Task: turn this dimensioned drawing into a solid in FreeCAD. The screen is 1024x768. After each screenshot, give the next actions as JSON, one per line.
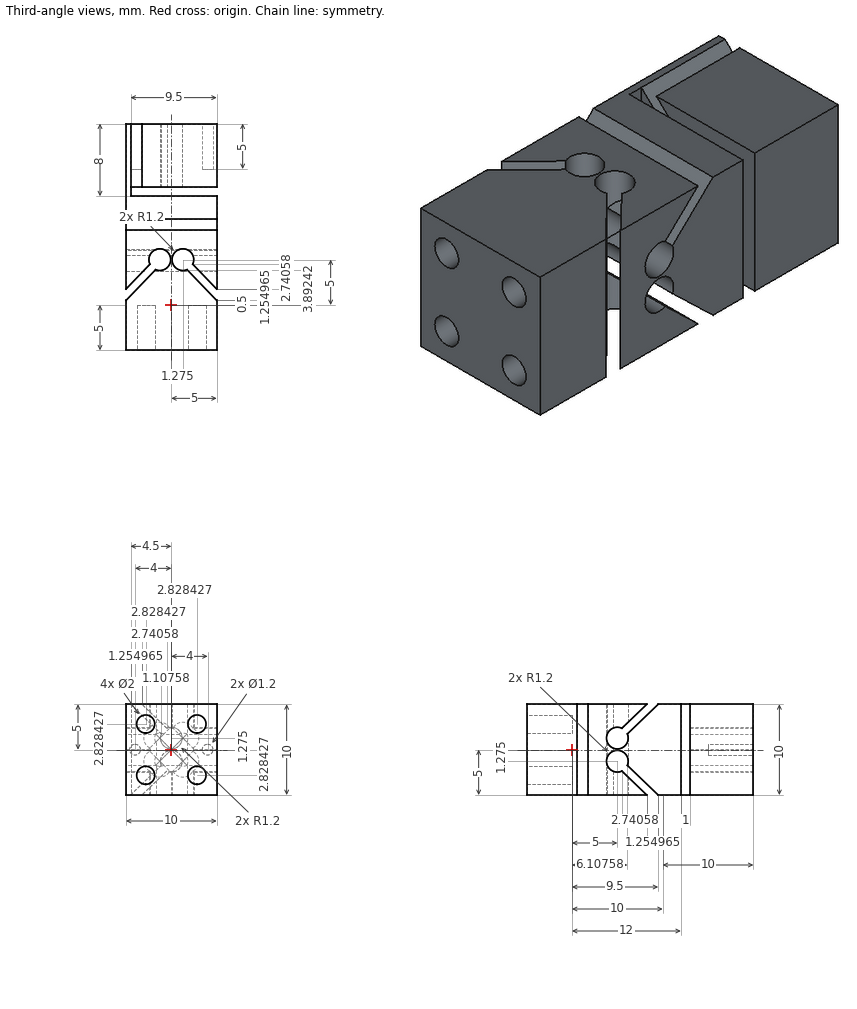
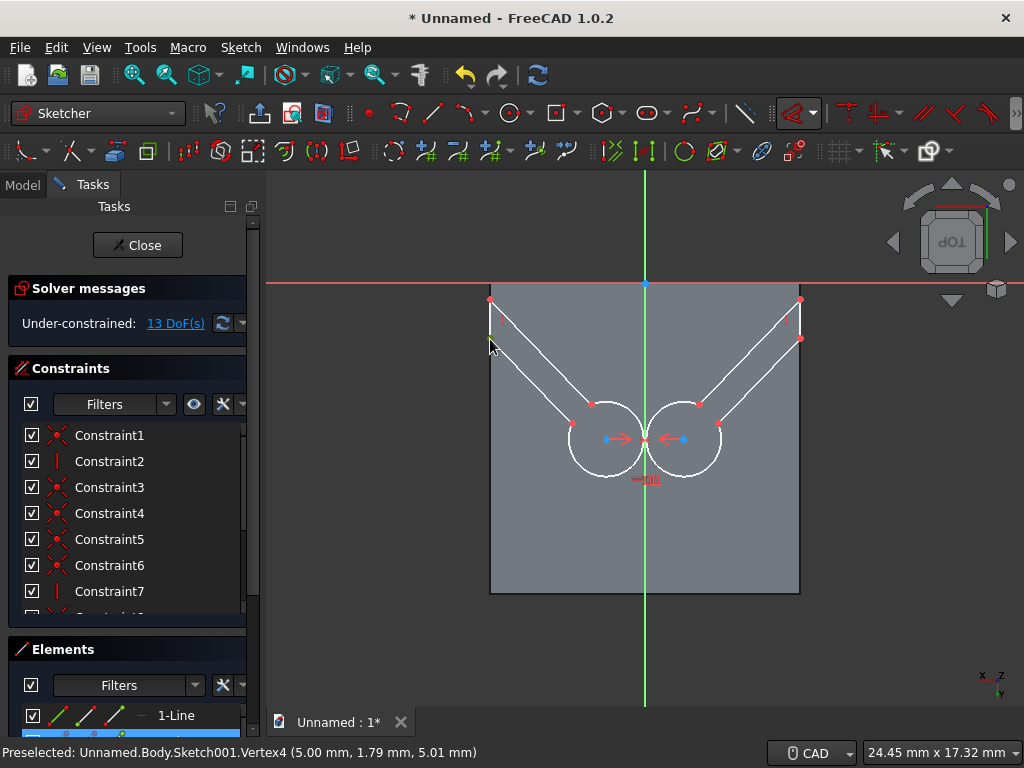
{"action": "left_click", "coordinate": [800, 339]}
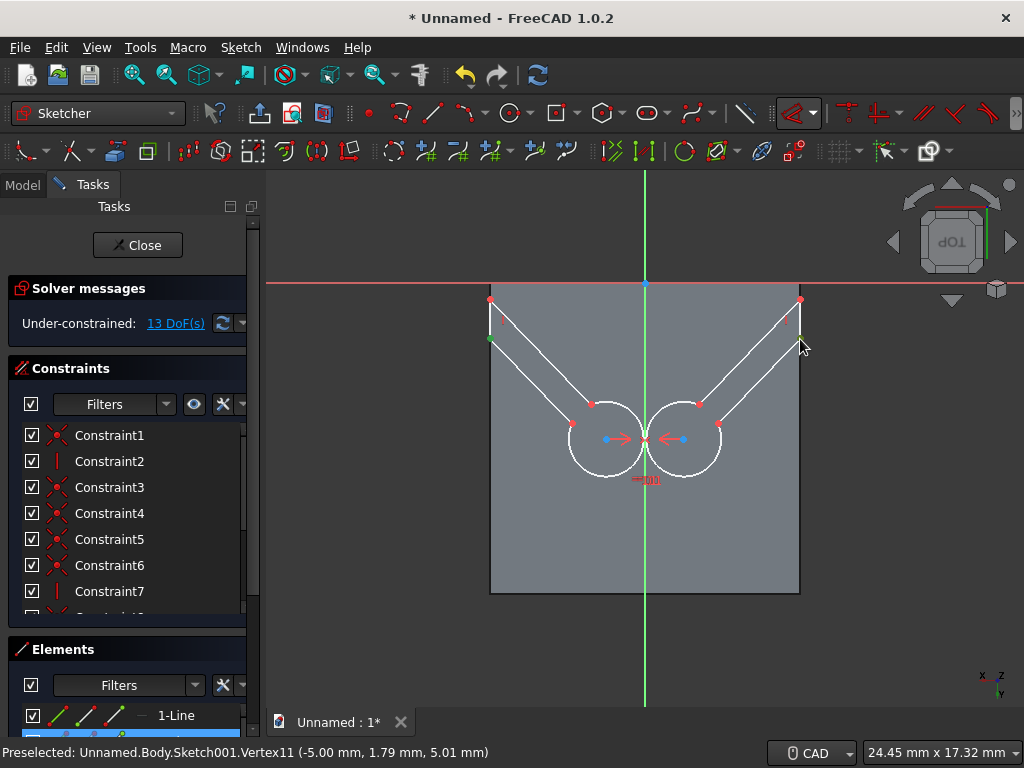
{"action": "left_click", "coordinate": [645, 645]}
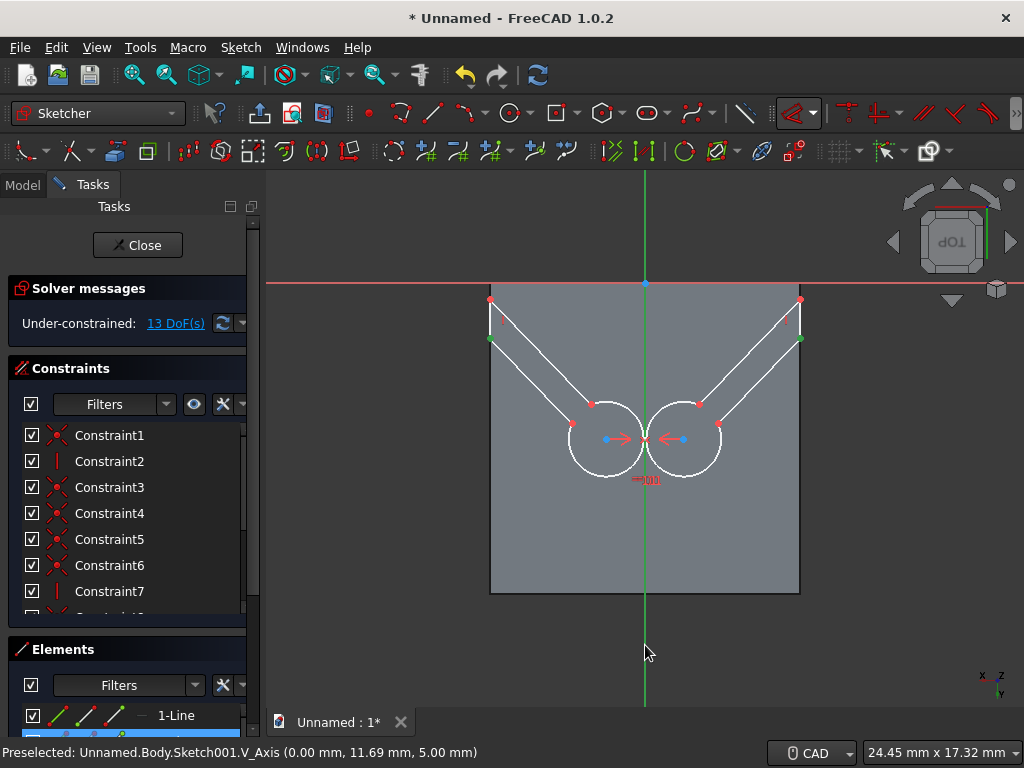
{"action": "key", "text": "s"}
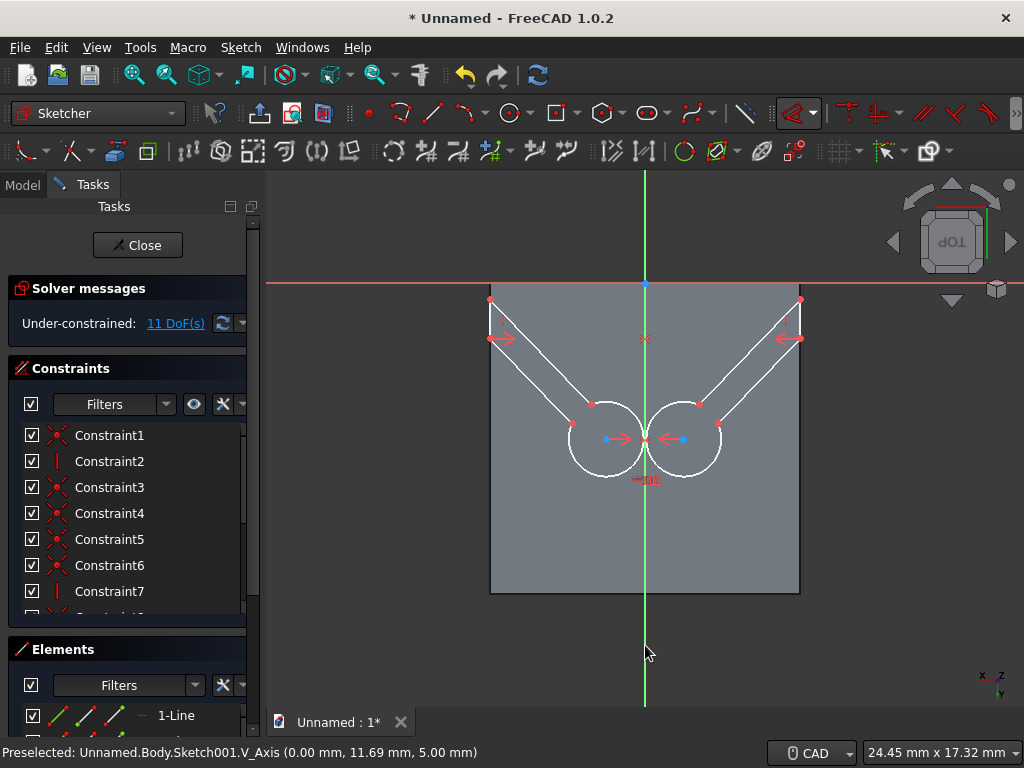
{"action": "left_click", "coordinate": [594, 475]}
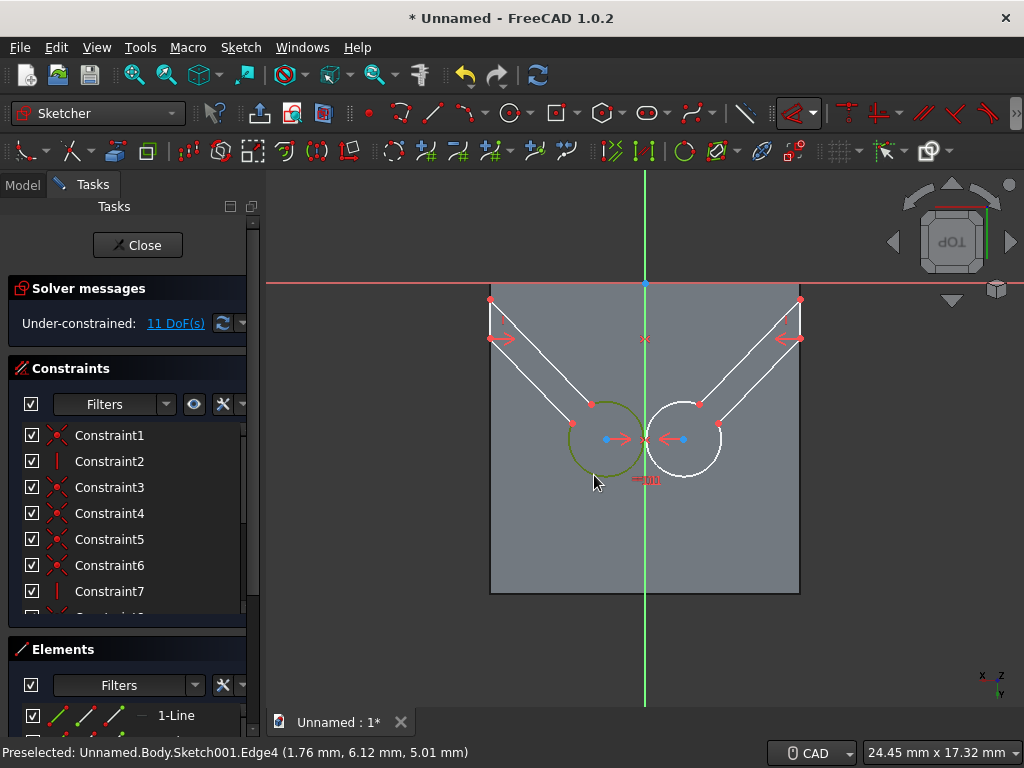
{"action": "key", "text": "k r"}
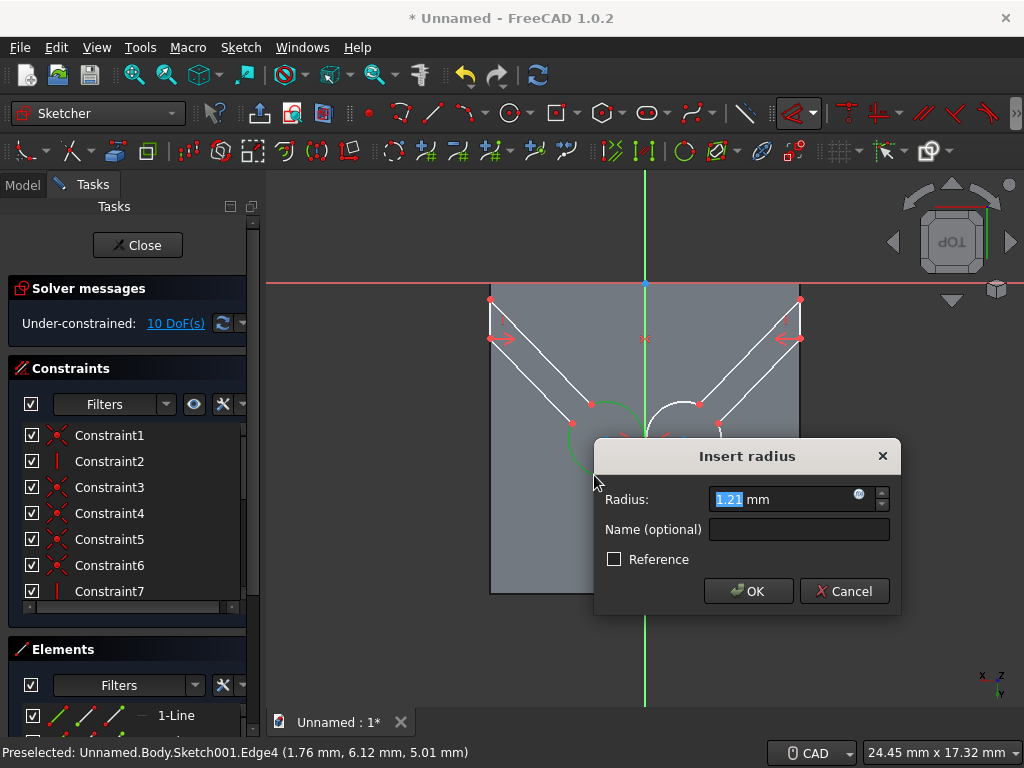
{"action": "type", "text": "1.2"}
{"action": "key", "text": "Return"}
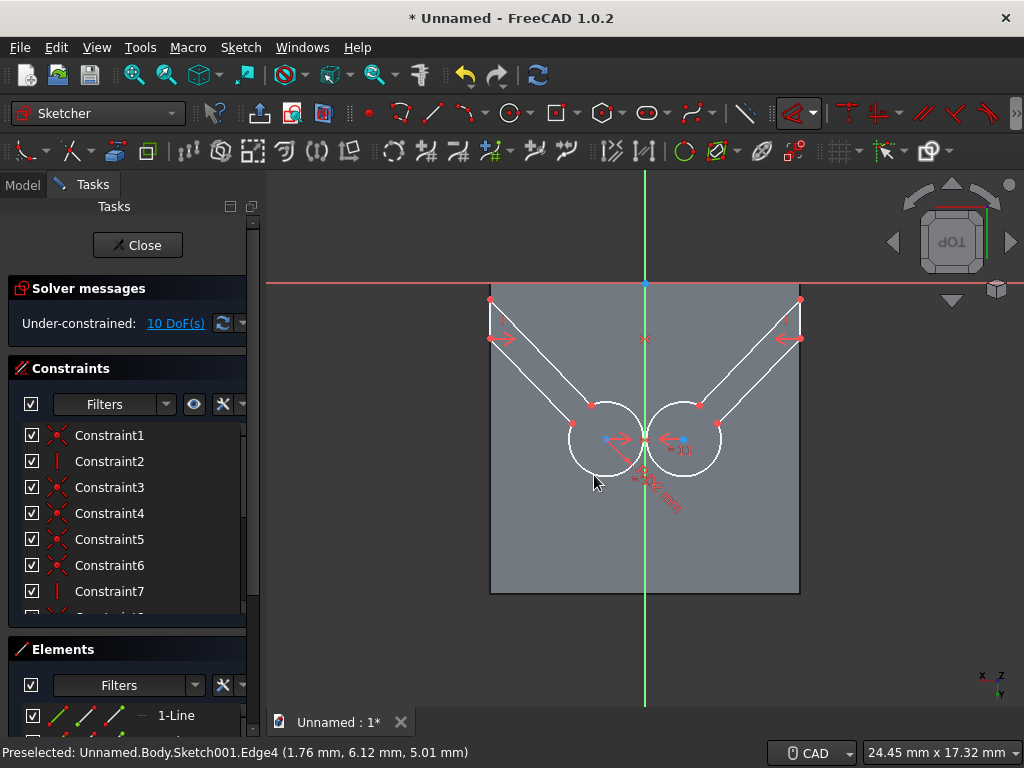
{"action": "left_click", "coordinate": [490, 300]}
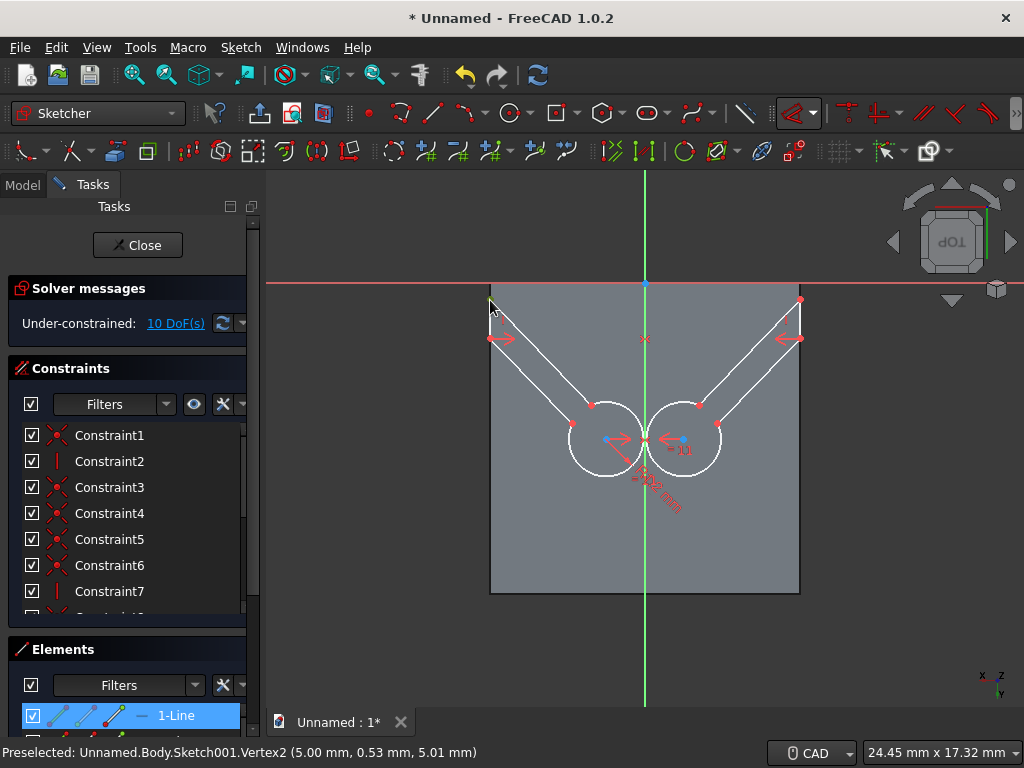
{"action": "key", "text": "l"}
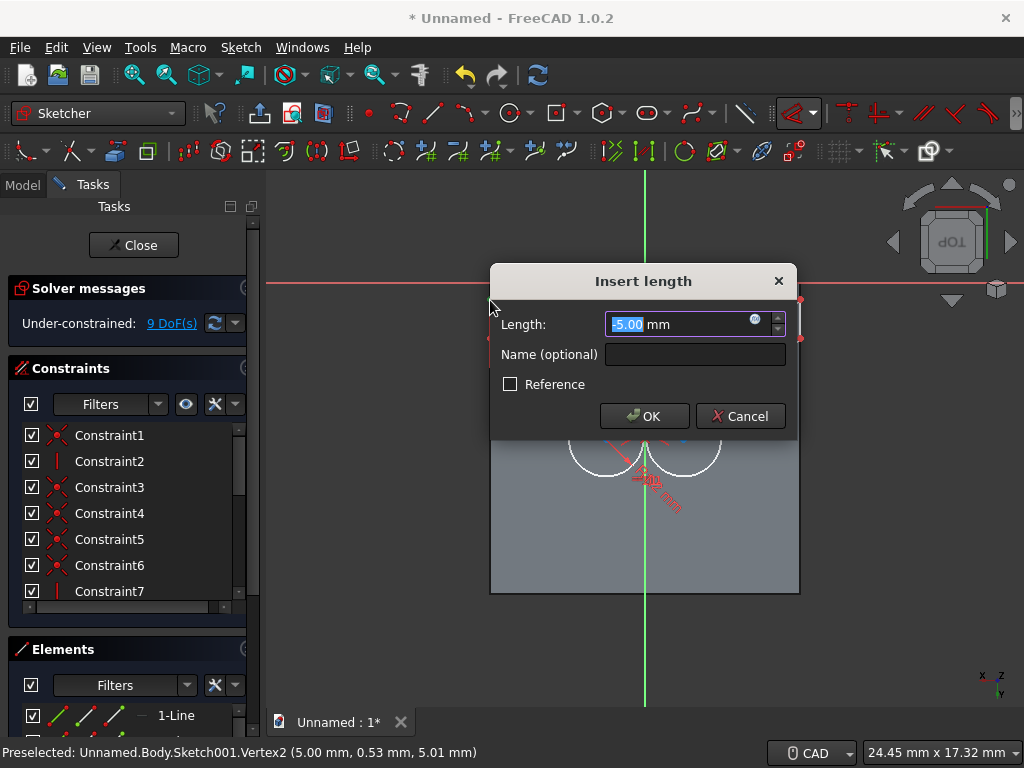
{"action": "type", "text": "-5"}
{"action": "key", "text": "Return"}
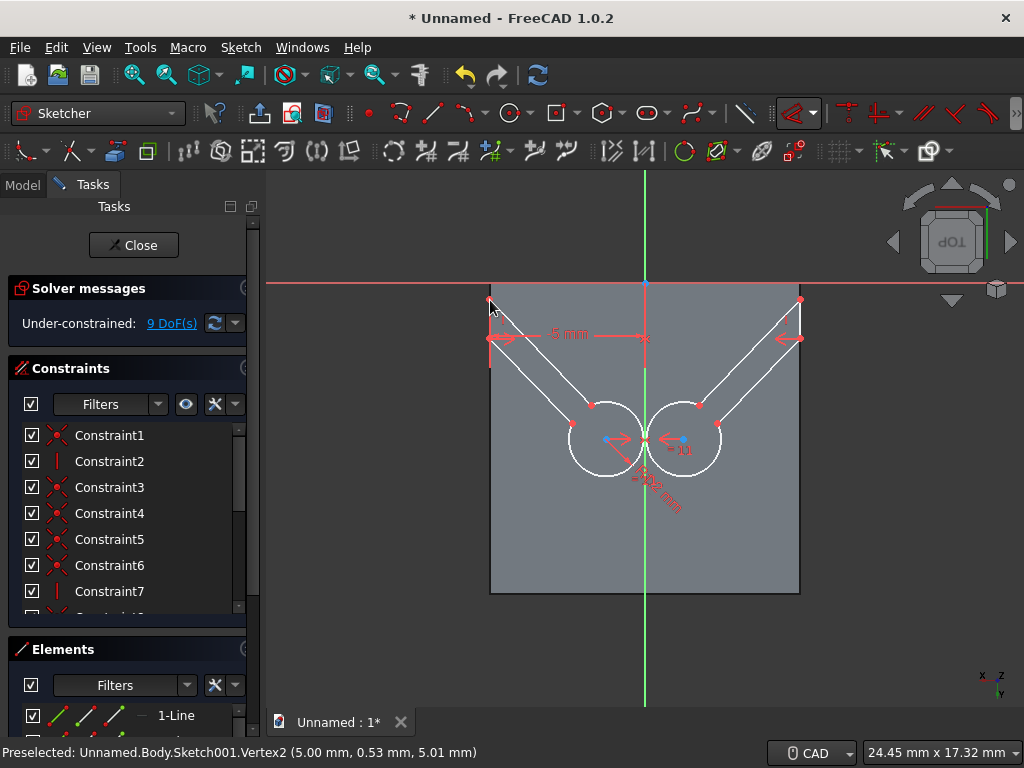
{"action": "left_click", "coordinate": [606, 439]}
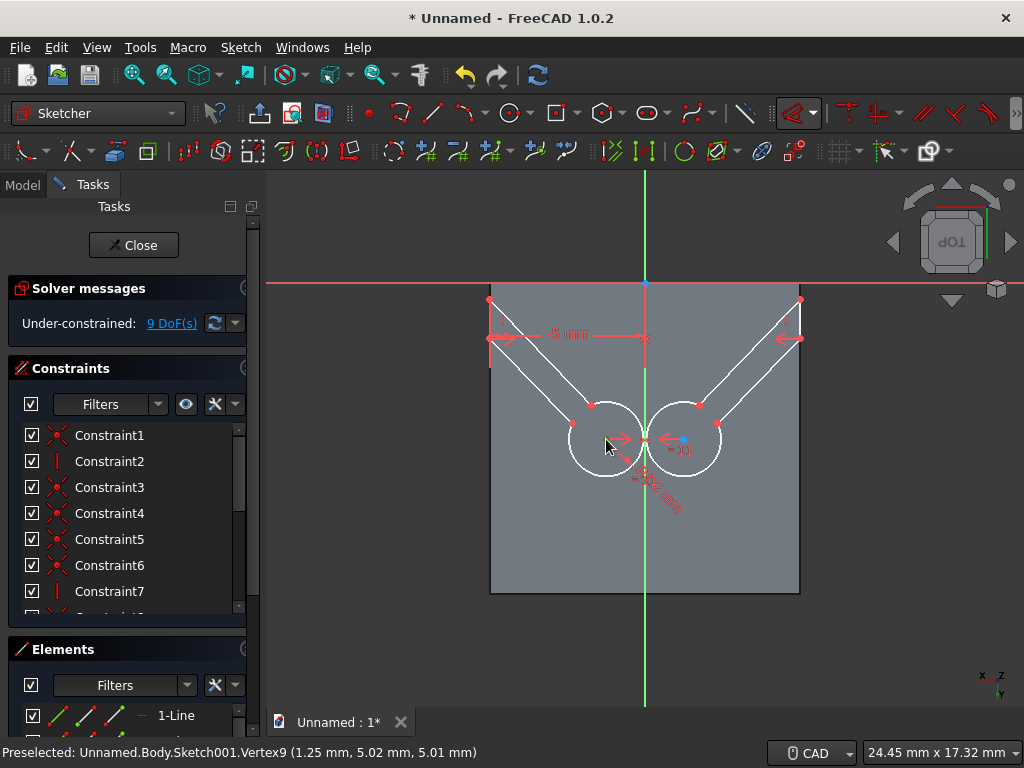
{"action": "left_click", "coordinate": [816, 114]}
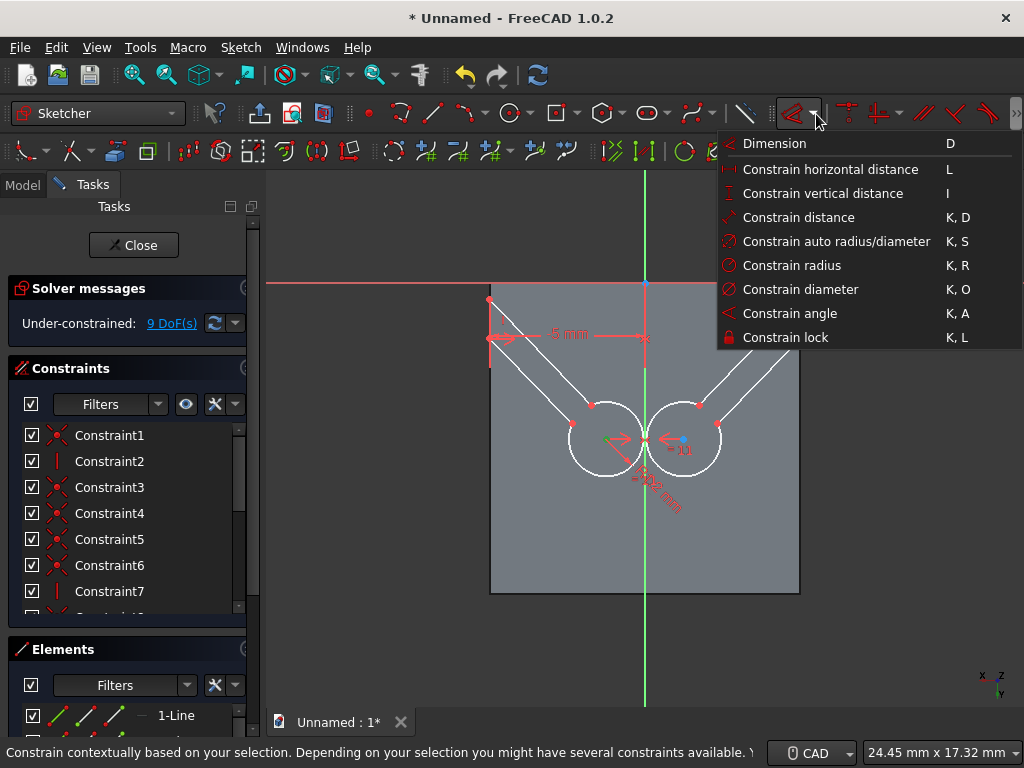
{"action": "left_click", "coordinate": [870, 193]}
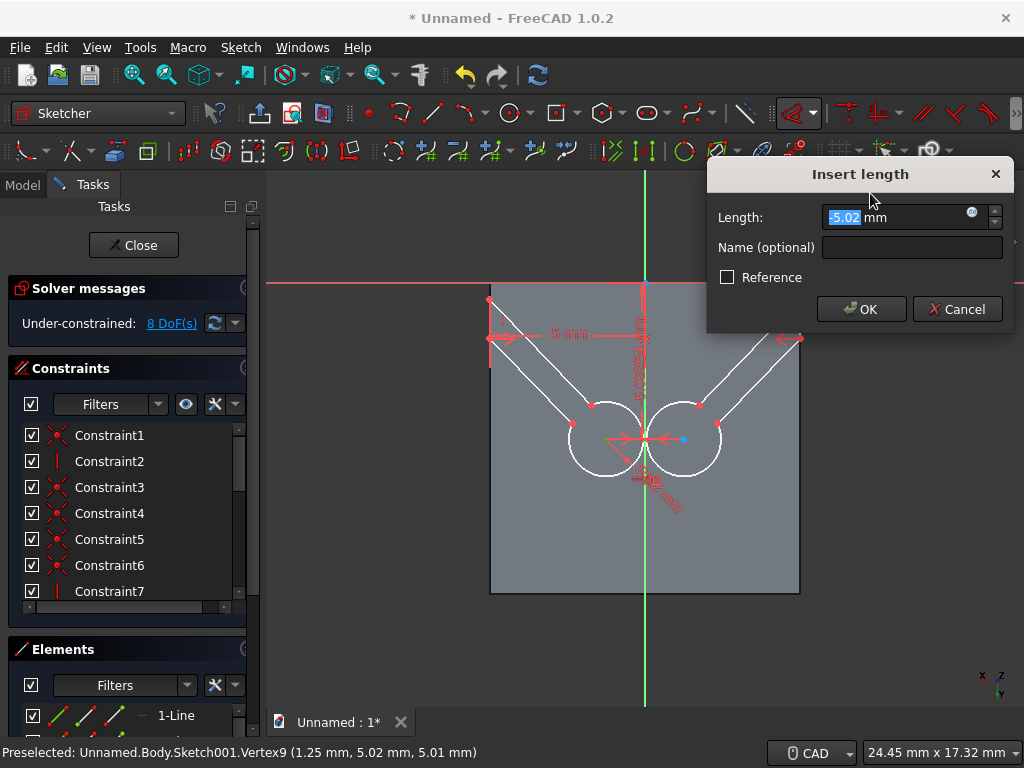
{"action": "type", "text": "-5"}
{"action": "key", "text": "Return"}